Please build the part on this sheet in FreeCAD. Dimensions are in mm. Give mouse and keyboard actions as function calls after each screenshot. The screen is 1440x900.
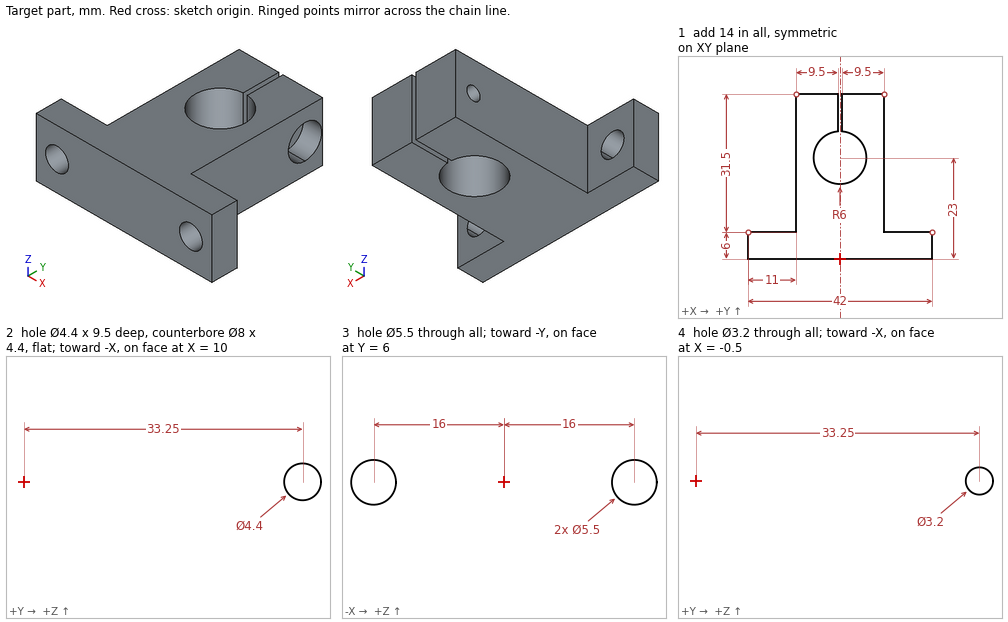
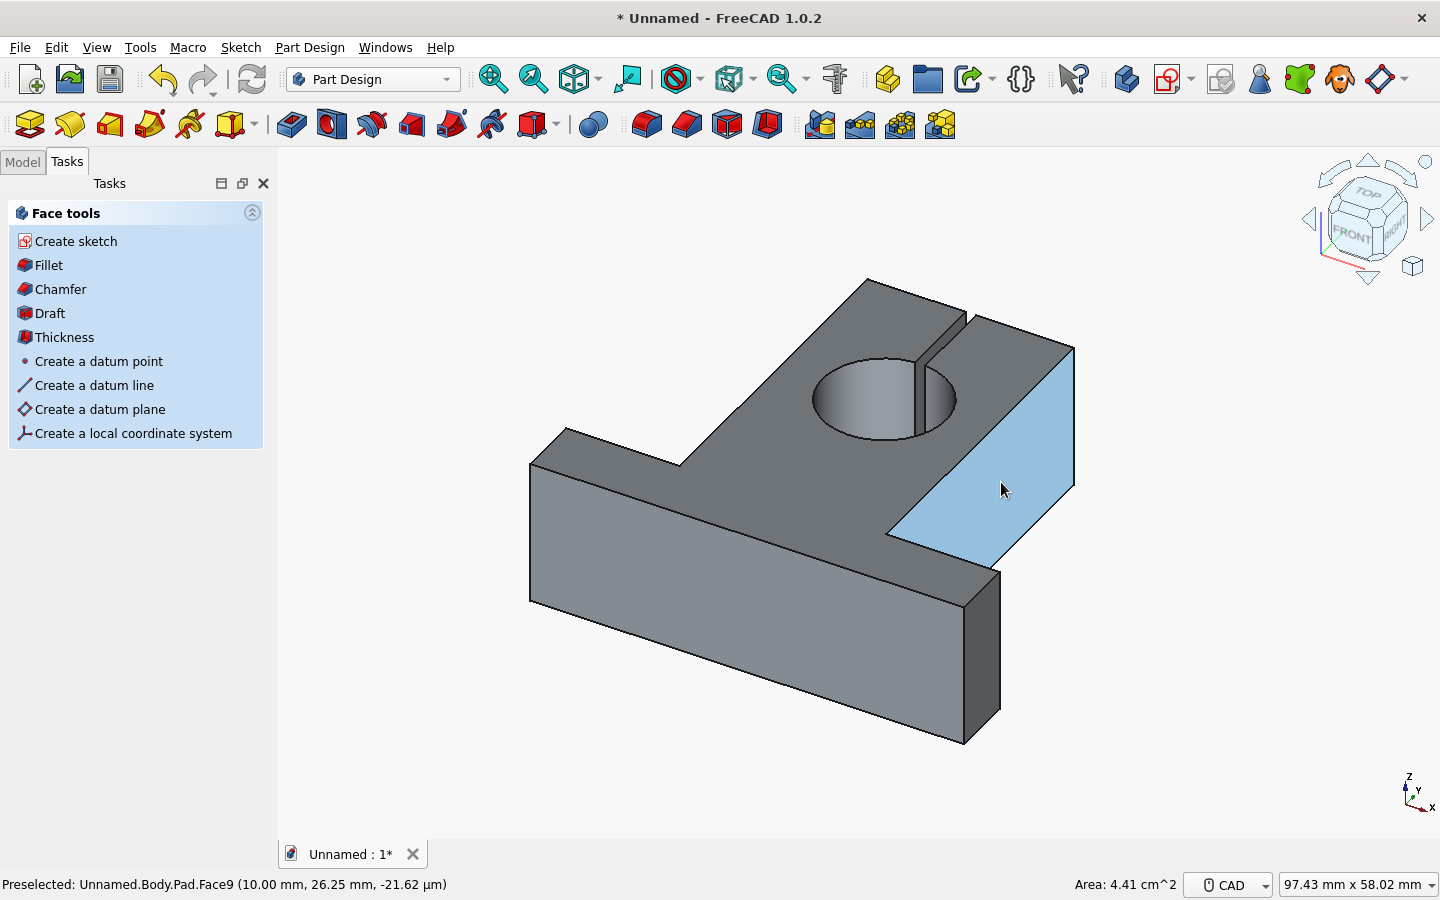
click(1168, 80)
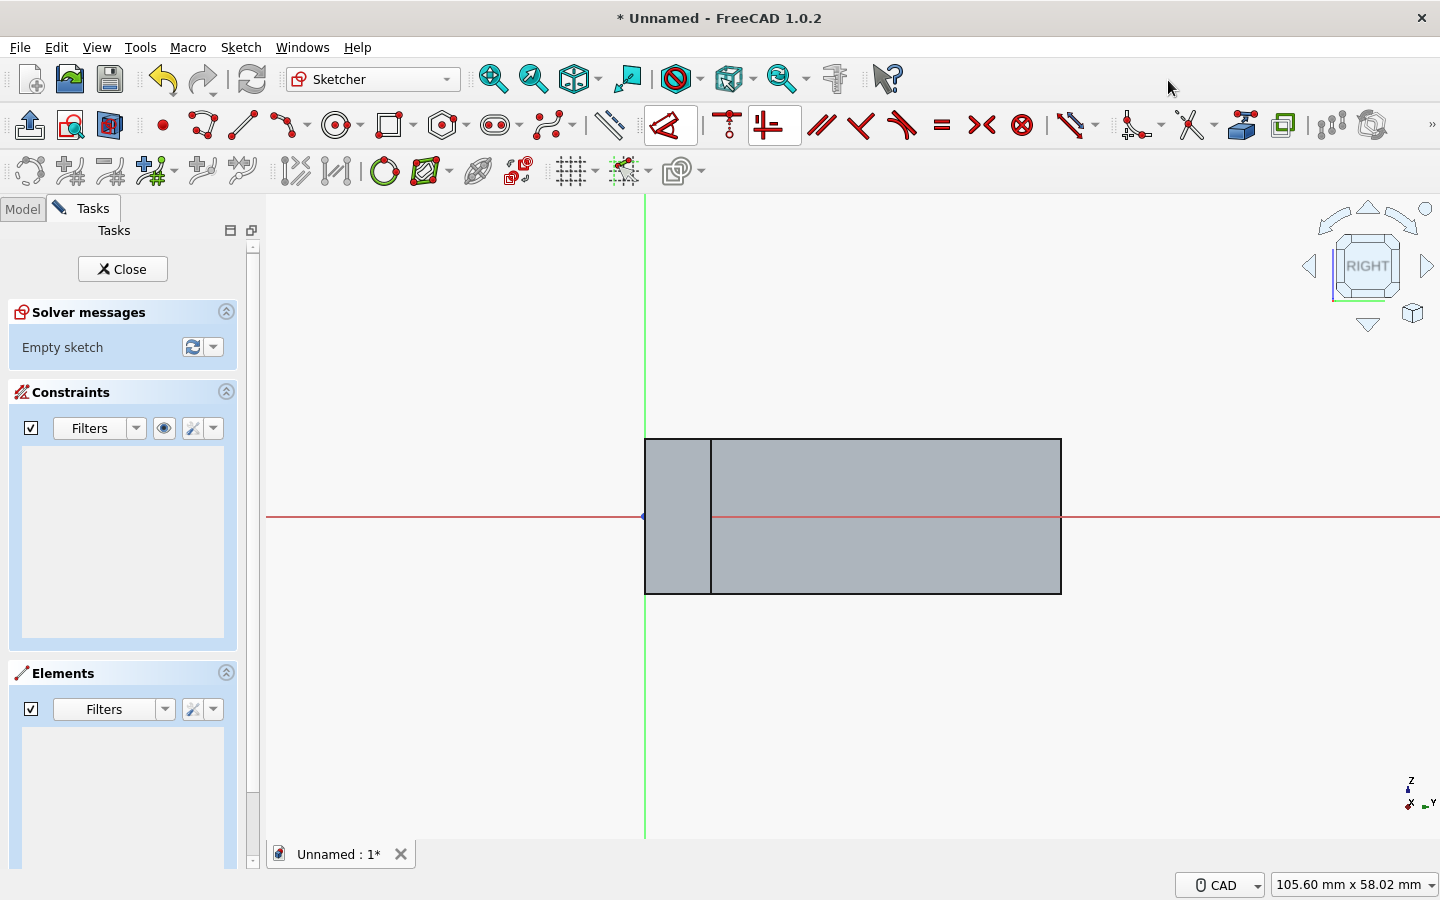
click(110, 126)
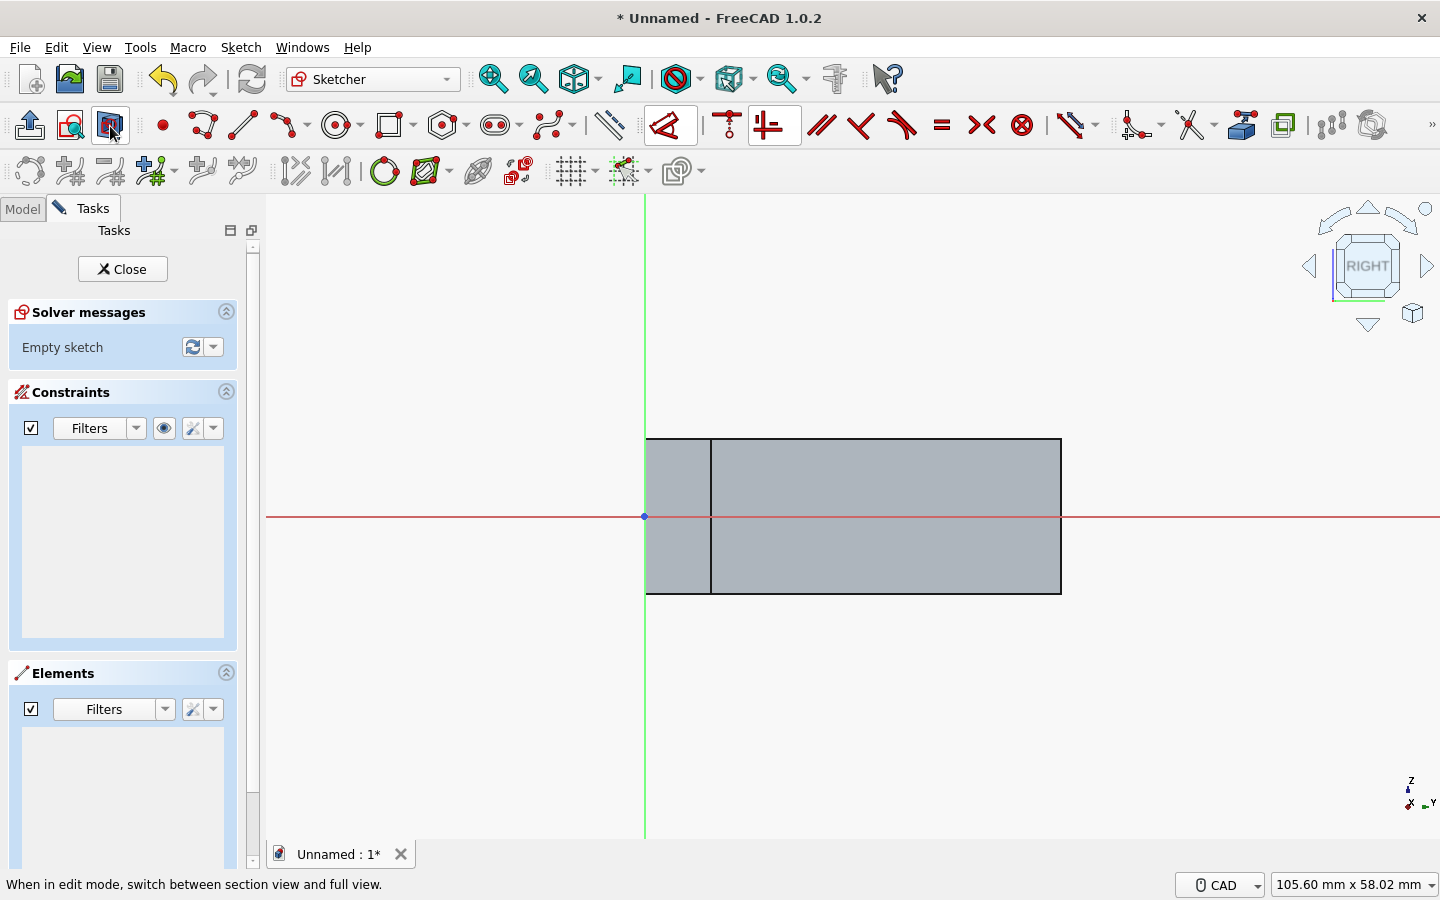
scroll(1043, 516, up, 11)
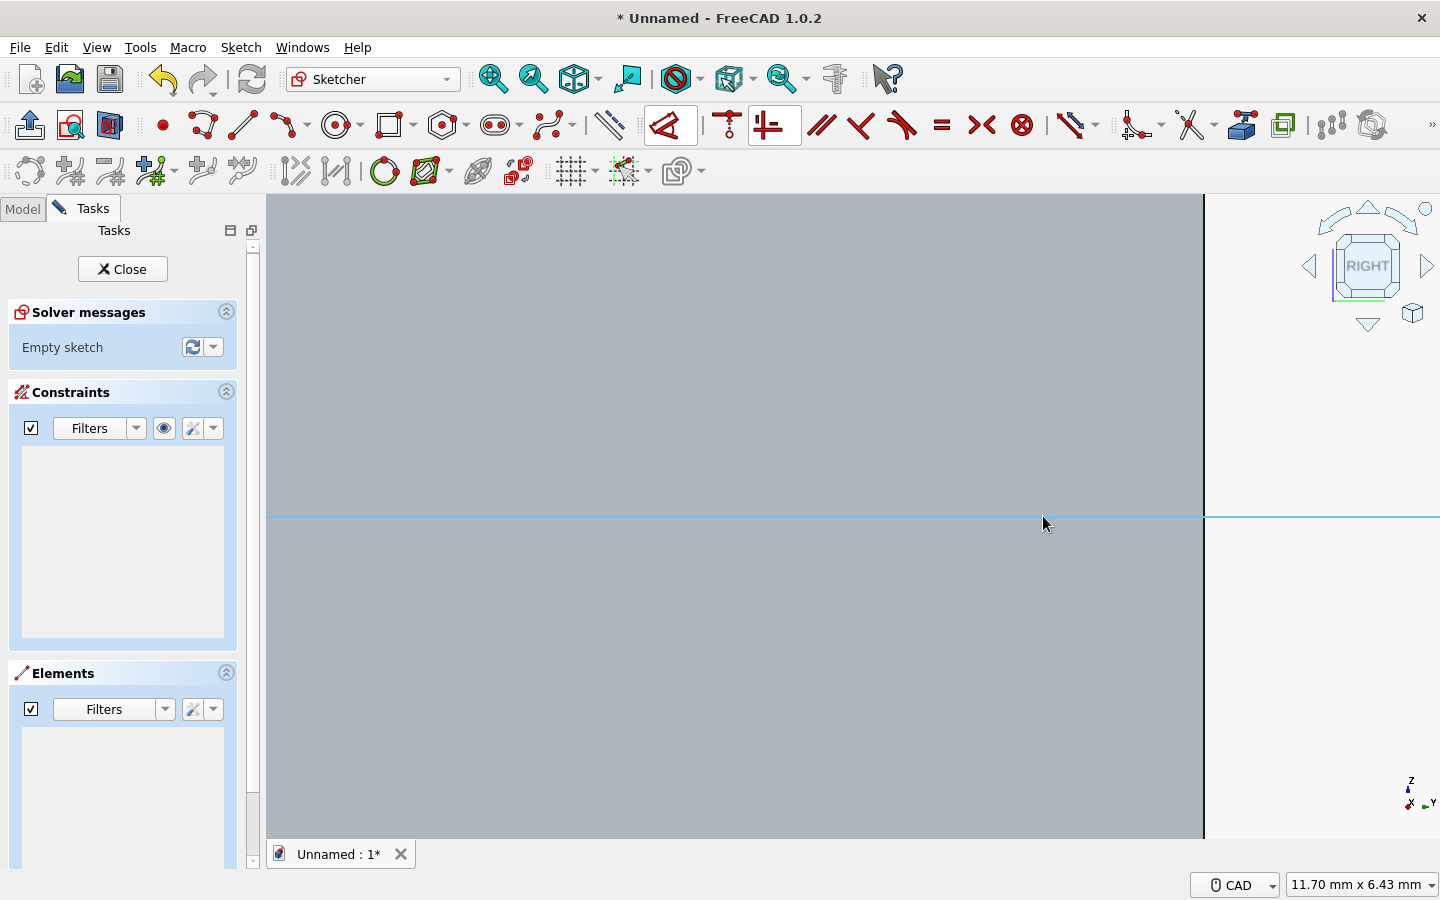
click(336, 126)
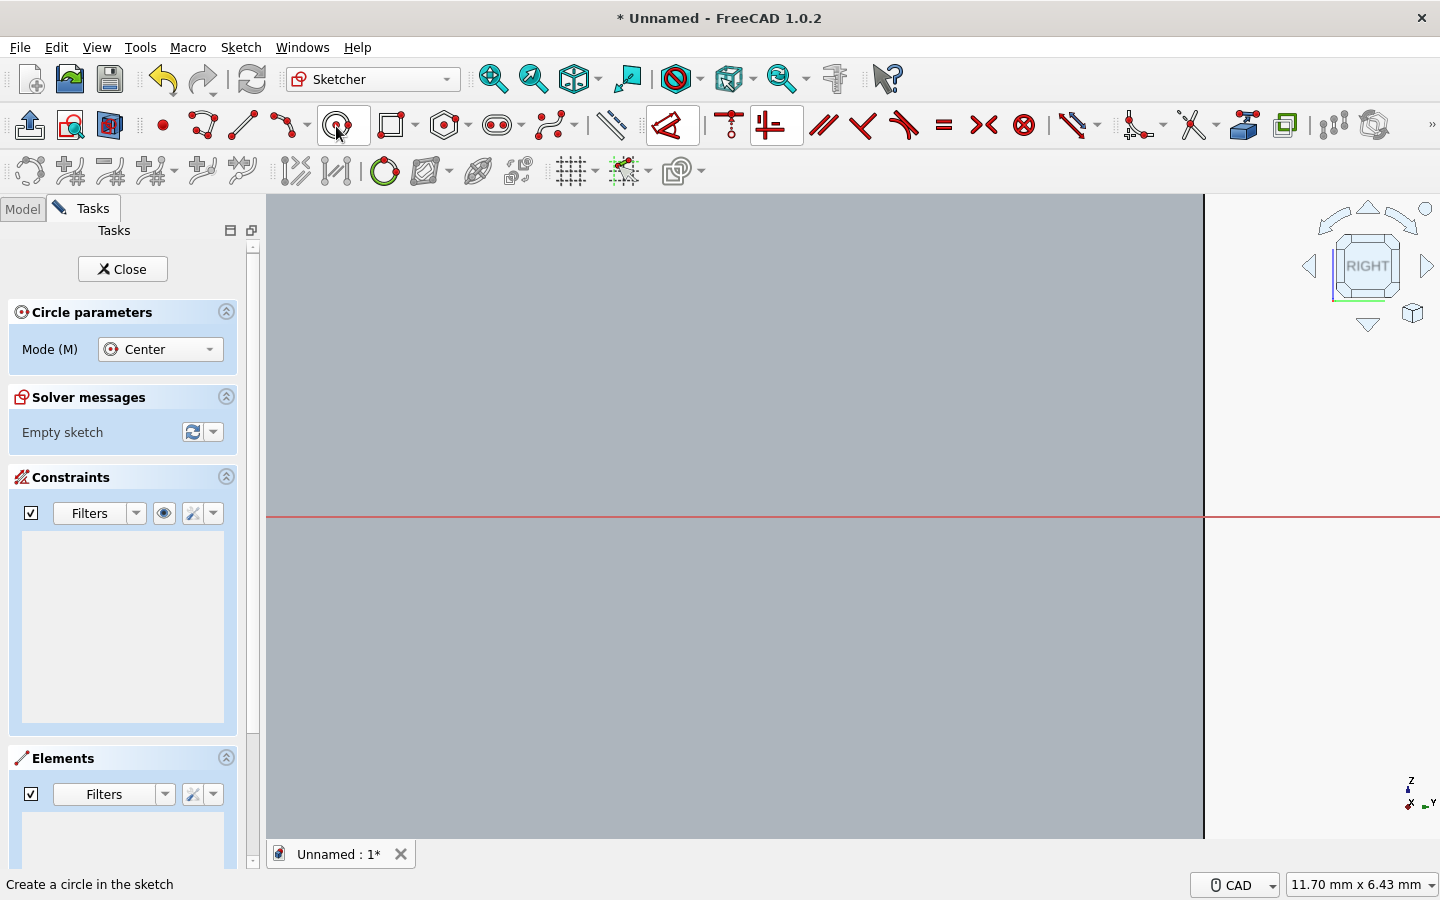
click(778, 516)
click(934, 360)
key(Escape)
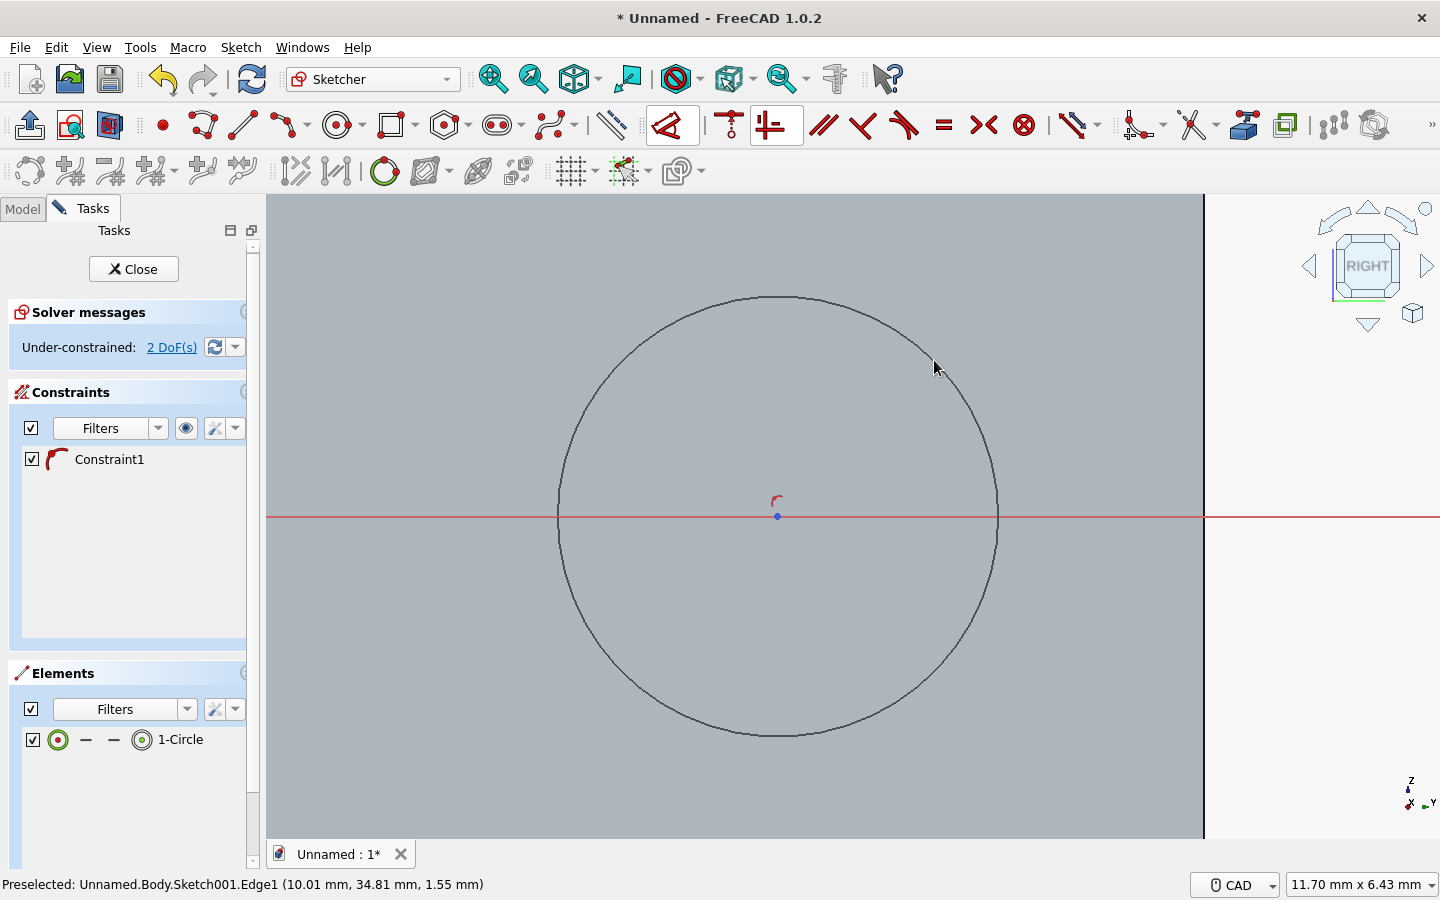
click(933, 360)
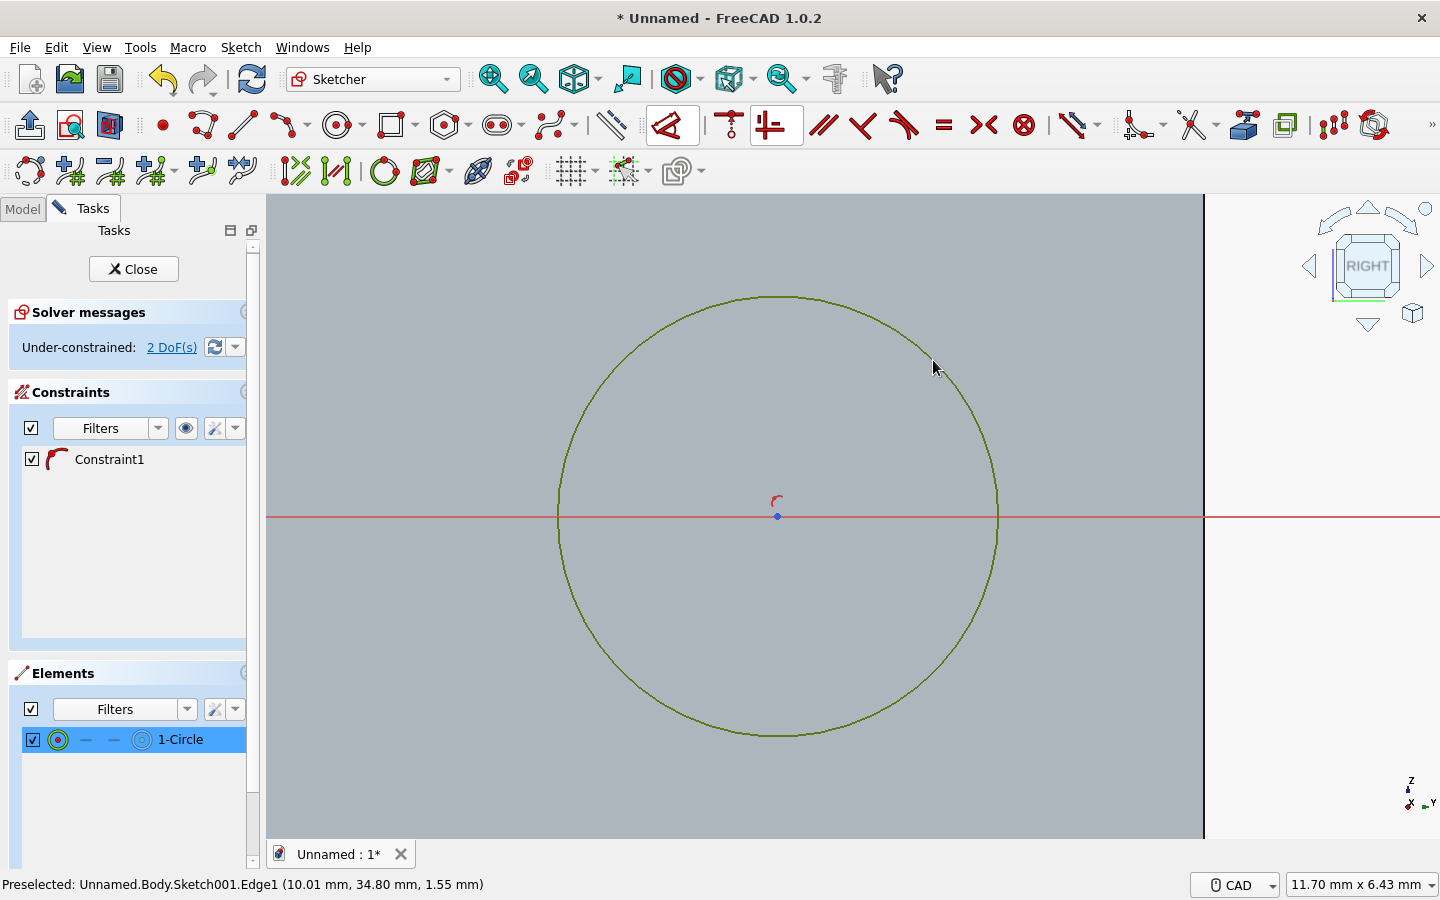
key(k)
key(o)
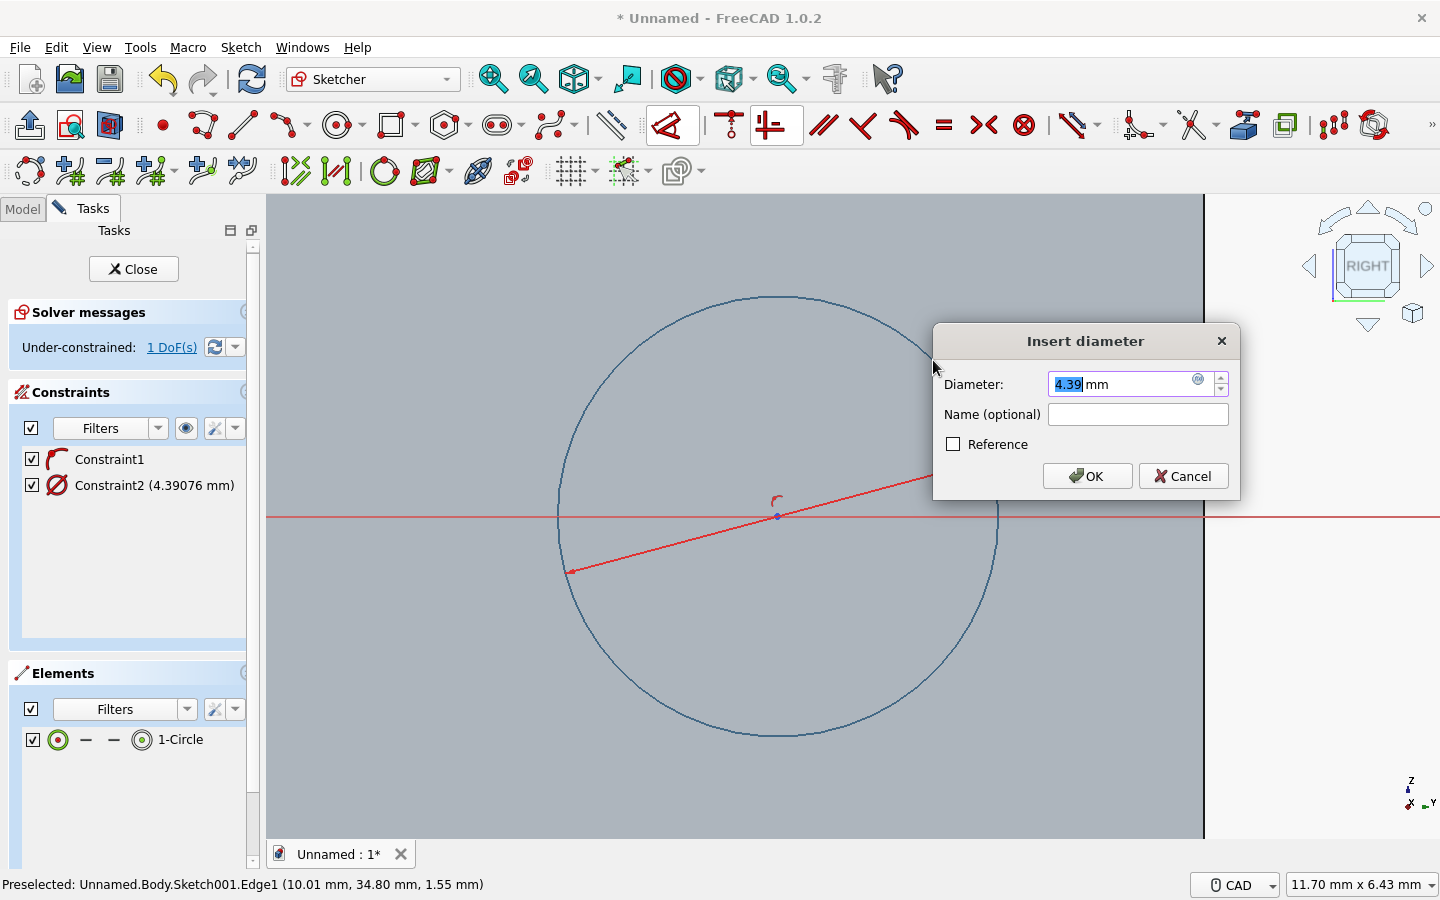
text(4.4)
key(Return)